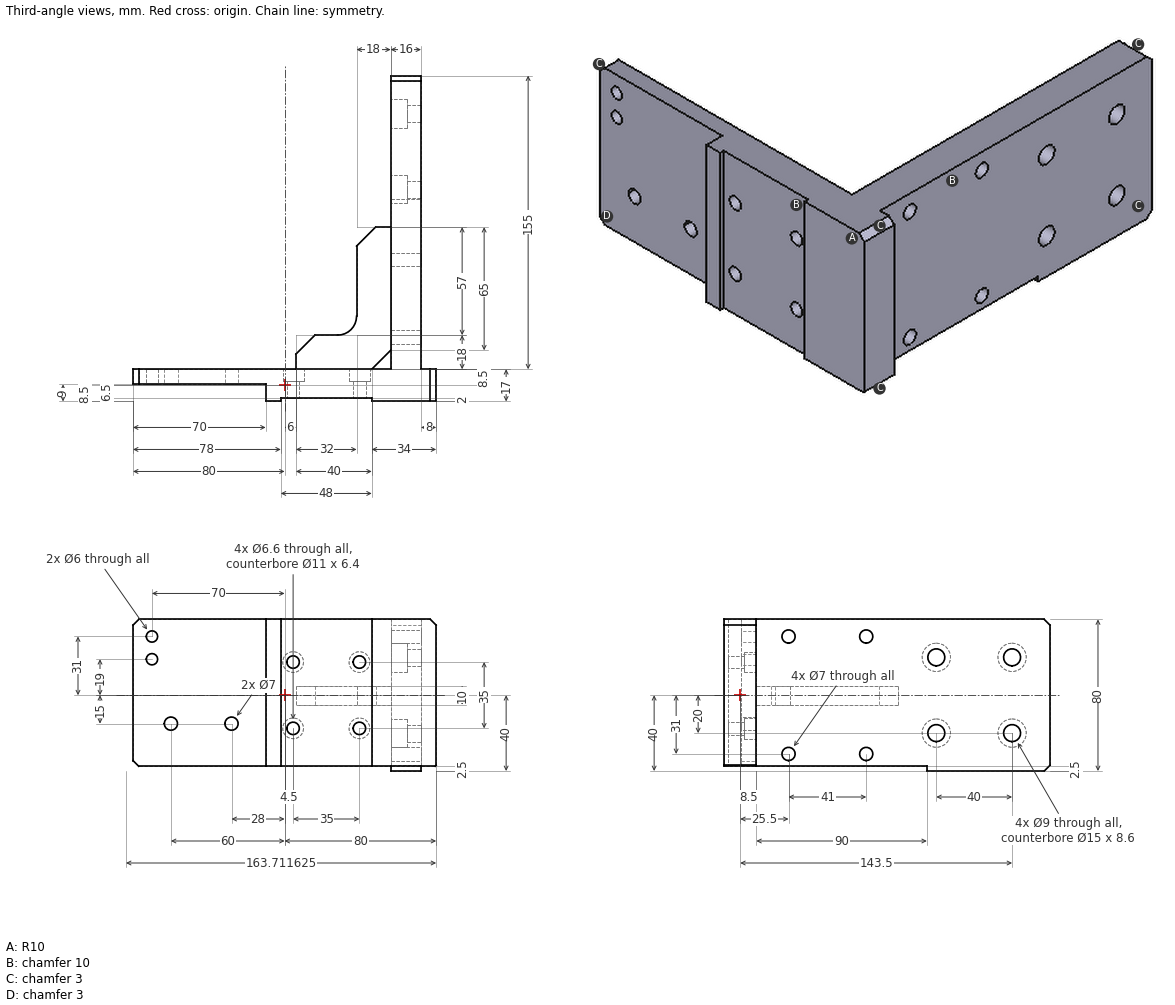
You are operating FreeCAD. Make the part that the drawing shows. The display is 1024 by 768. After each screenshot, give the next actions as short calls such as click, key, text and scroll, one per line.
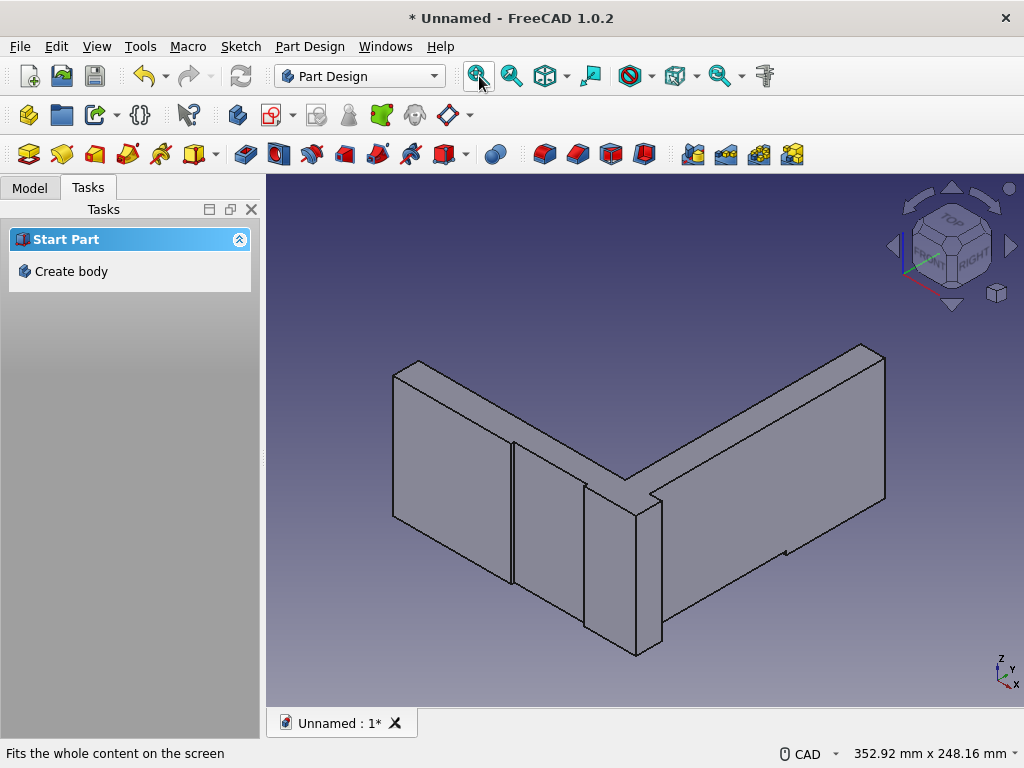
key(2)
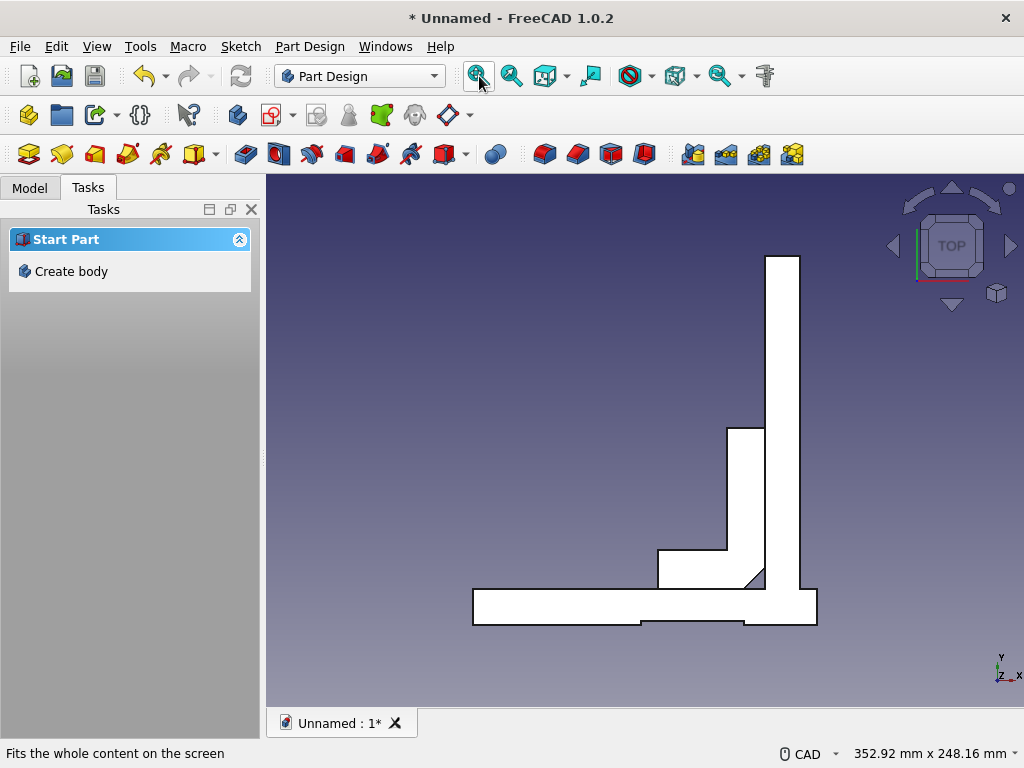
scroll(727, 549, up, 4)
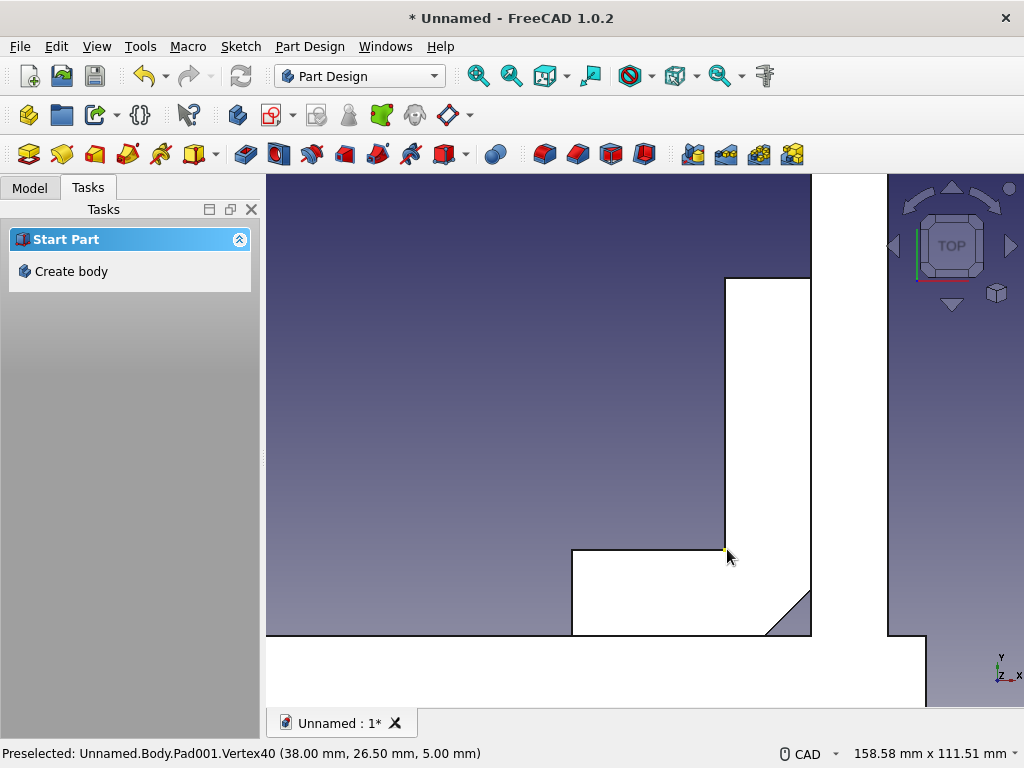
click(479, 76)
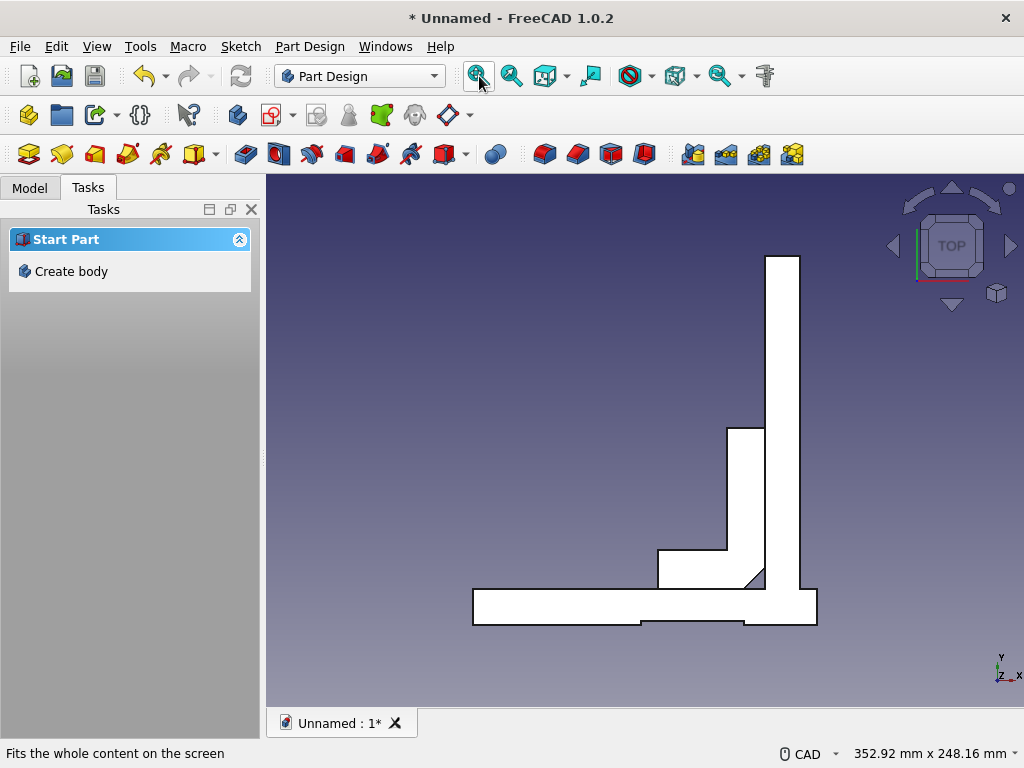
key(1)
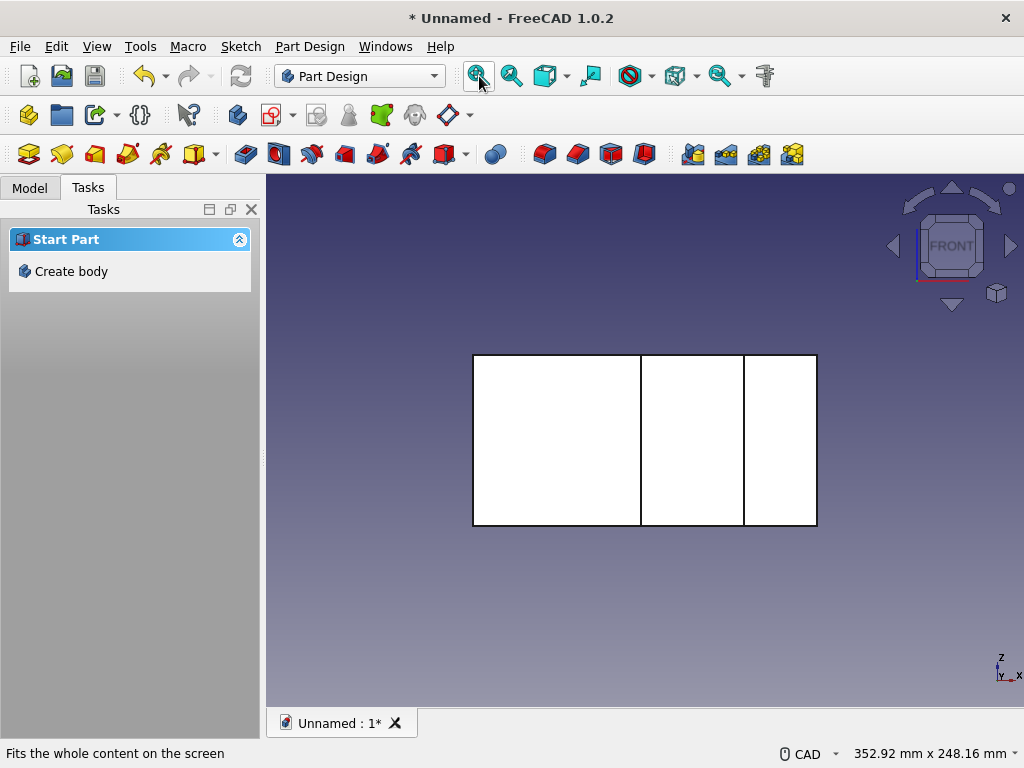
scroll(727, 440, up, 4)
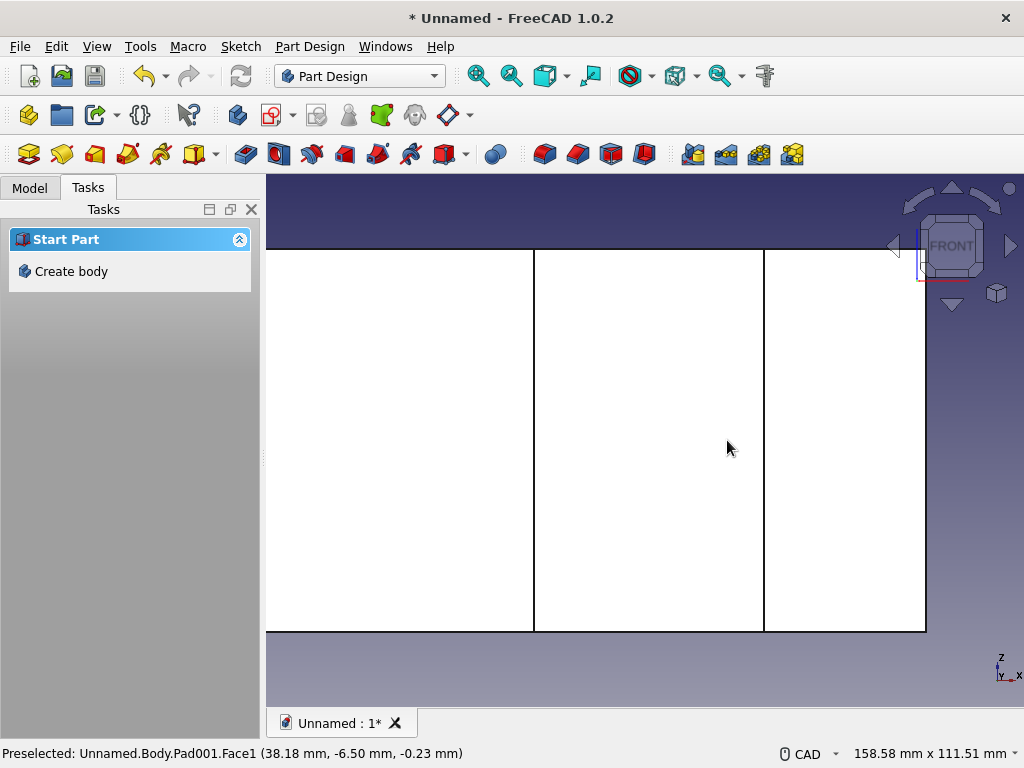
click(479, 76)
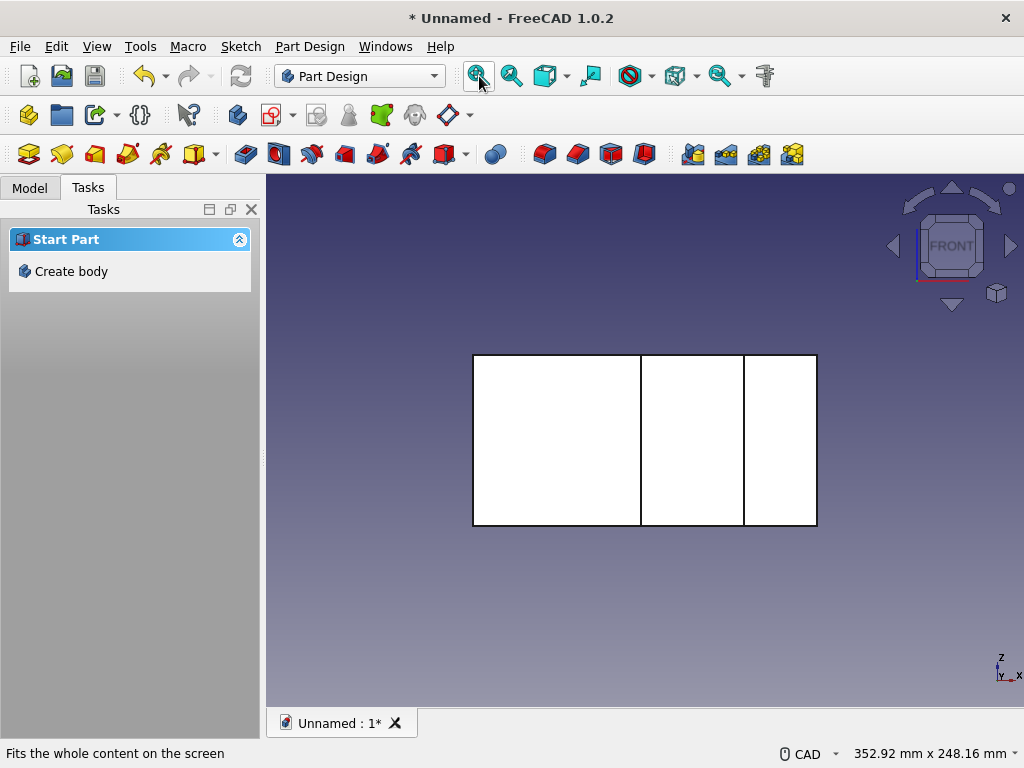
key(3)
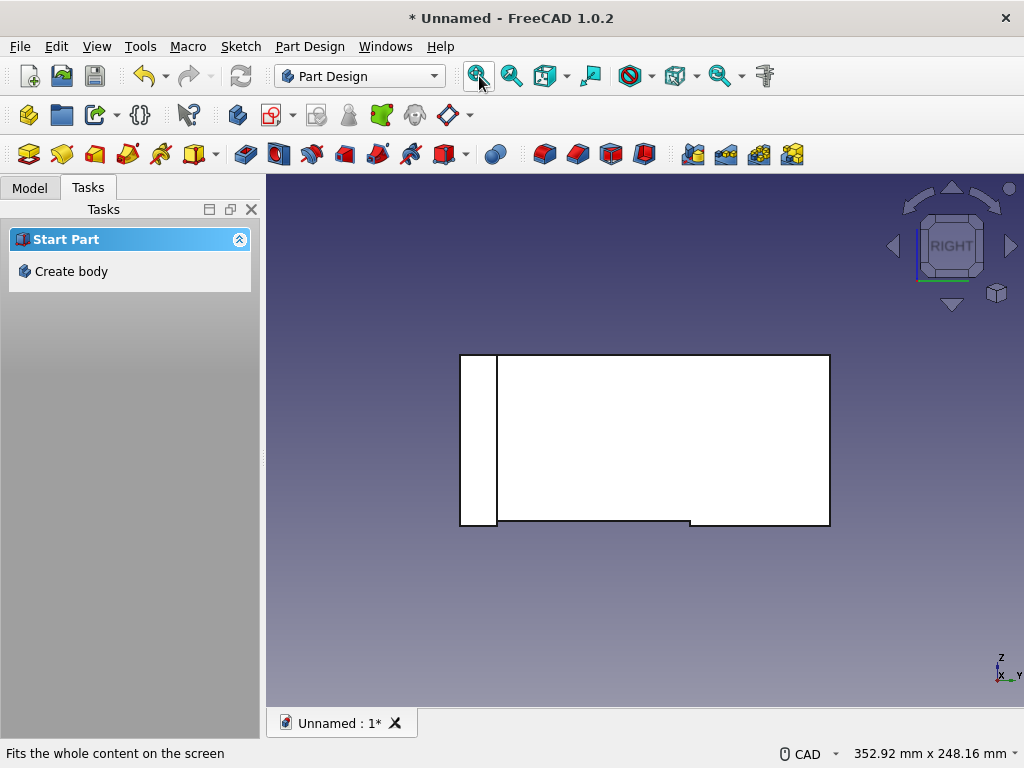
scroll(535, 439, up, 4)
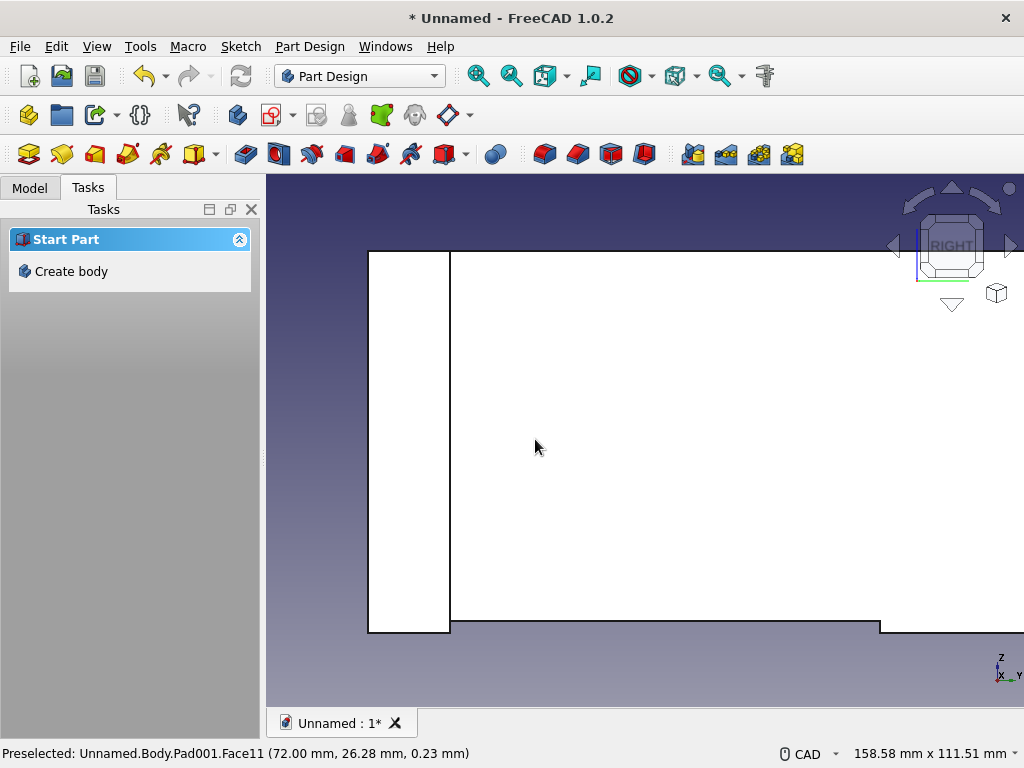
click(479, 76)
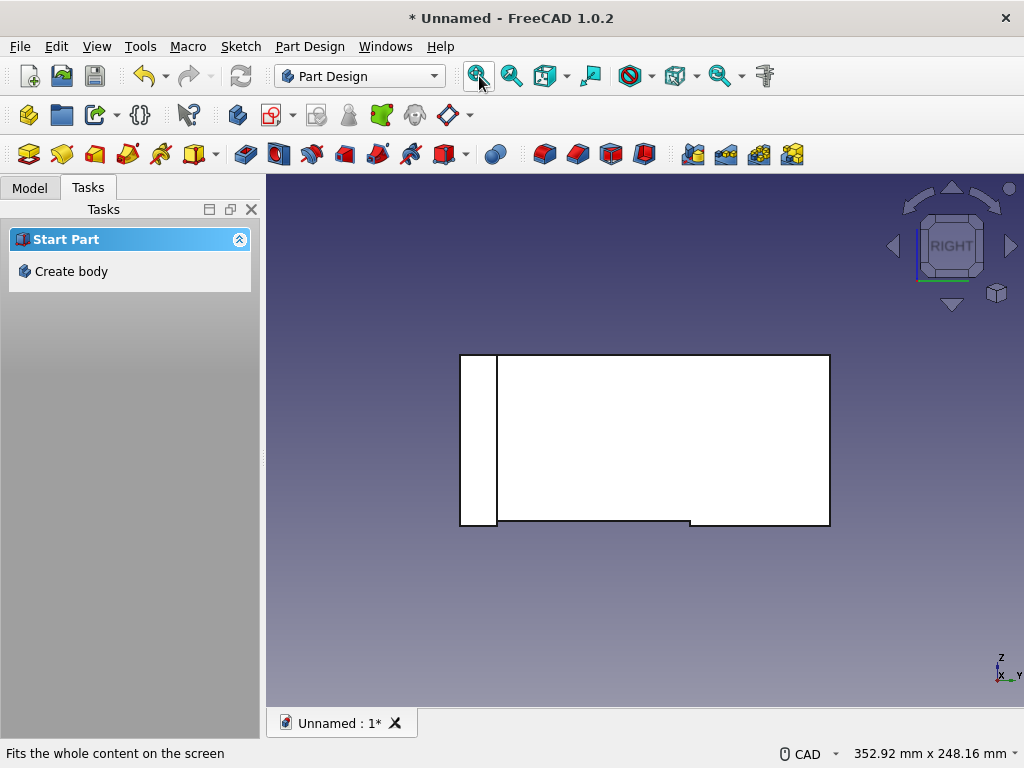
key(5)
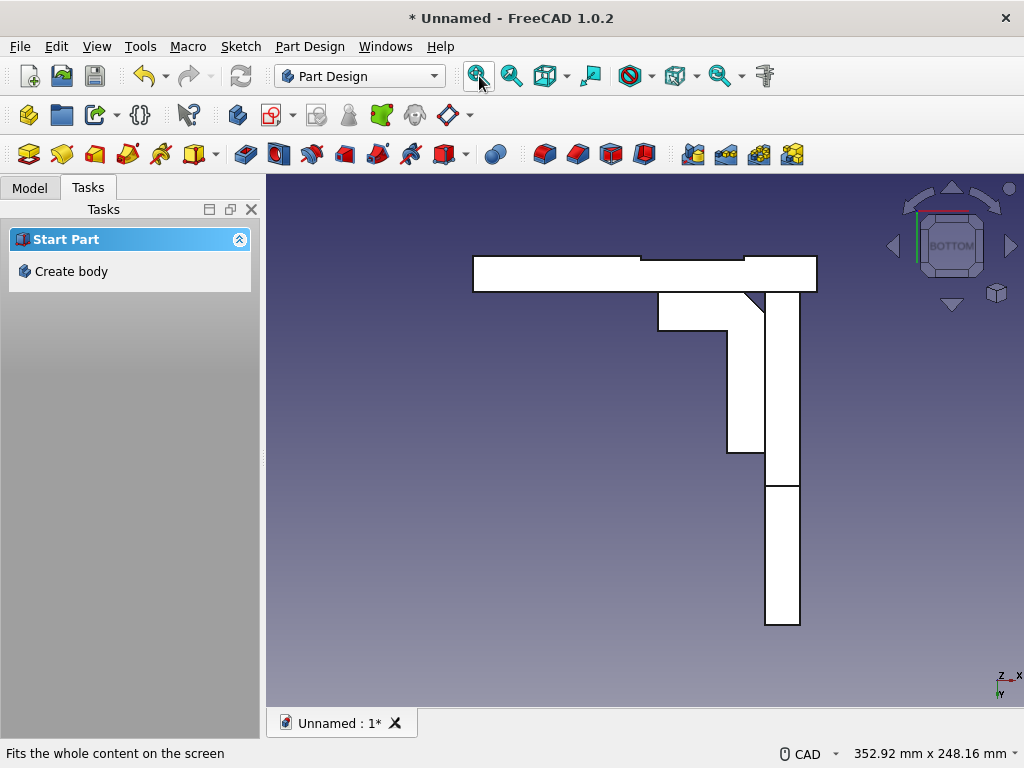
scroll(727, 330, up, 4)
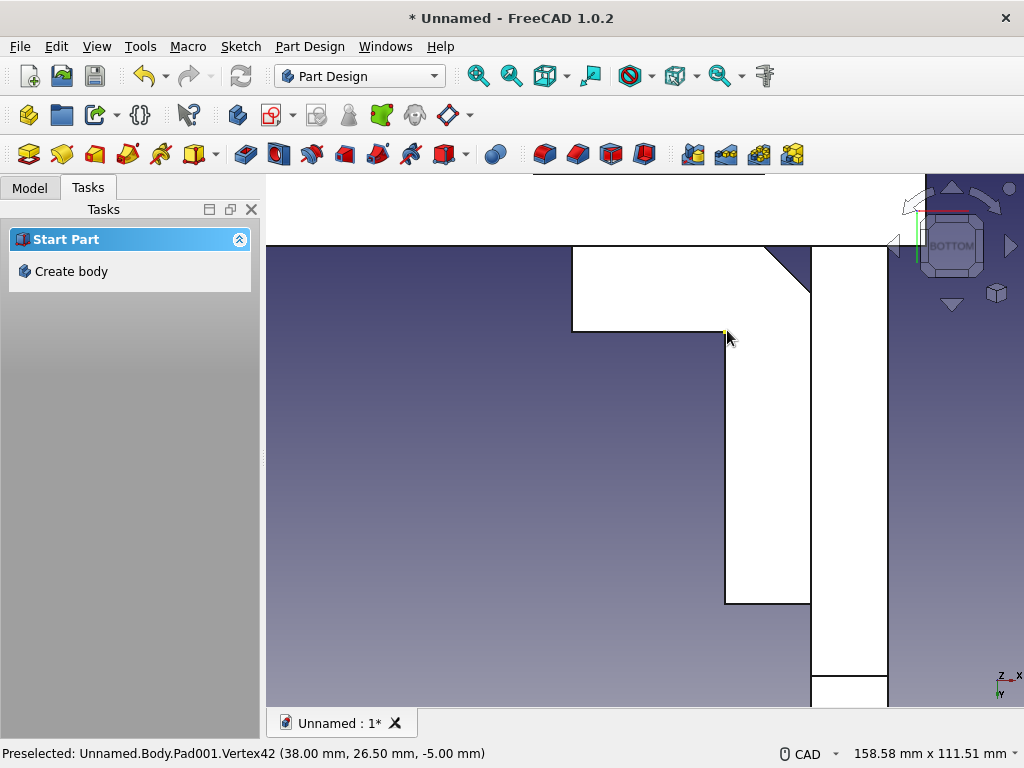
click(479, 76)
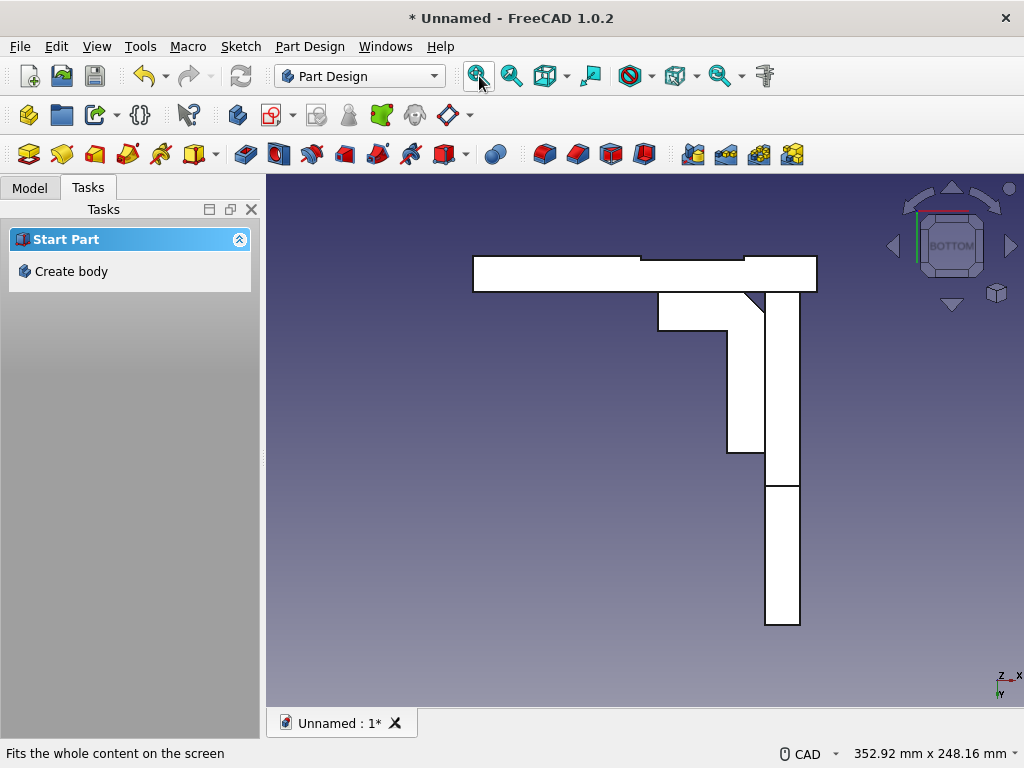
key(4)